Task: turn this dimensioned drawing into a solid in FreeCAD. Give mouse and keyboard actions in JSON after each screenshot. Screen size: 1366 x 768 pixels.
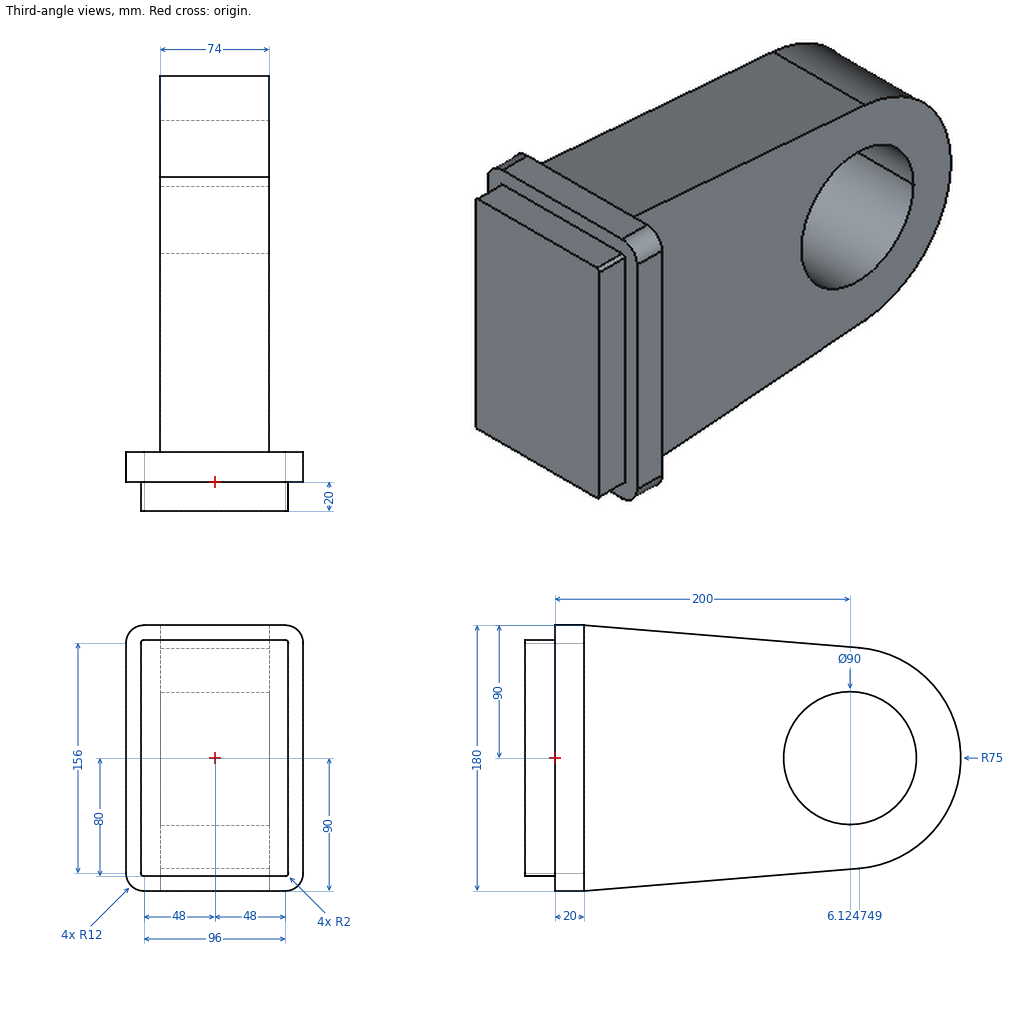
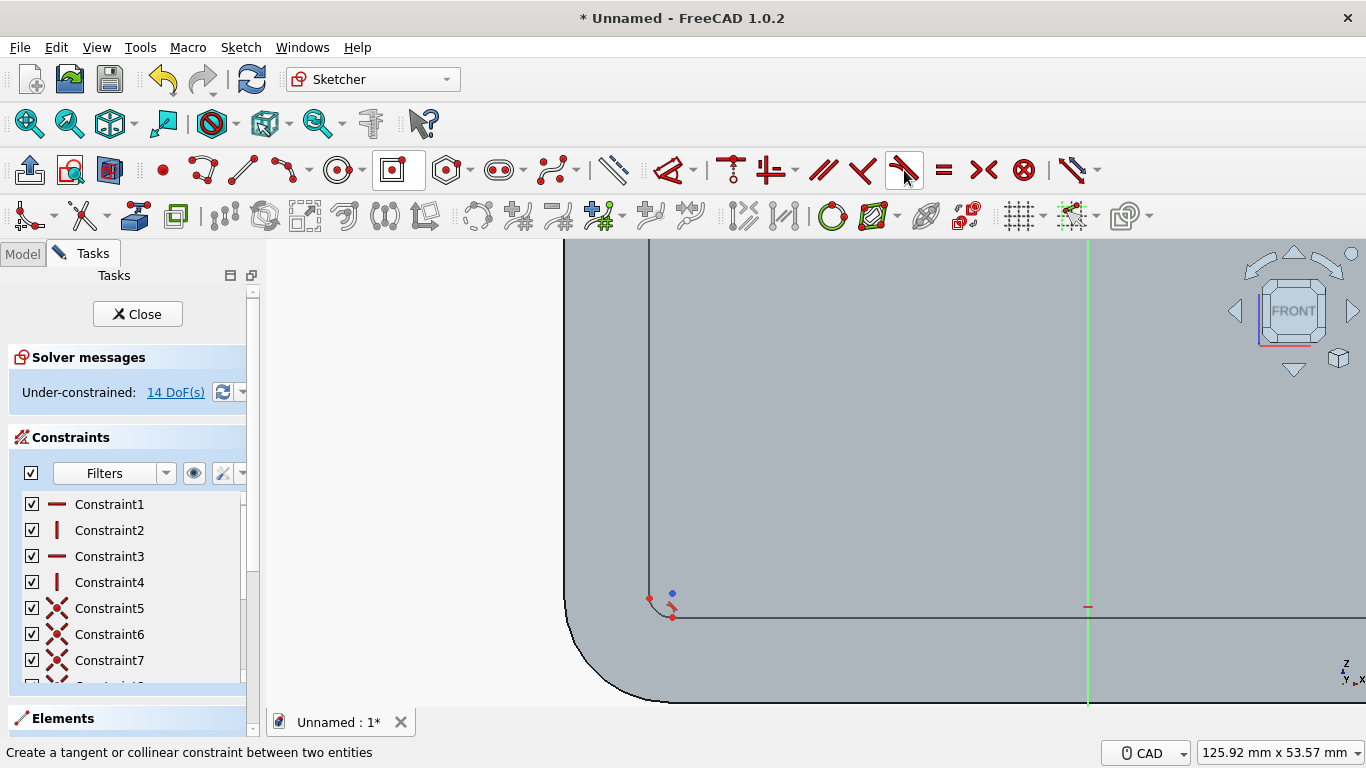
{"action": "scroll", "coordinate": [661, 614], "scroll_direction": "down", "scroll_amount": 8}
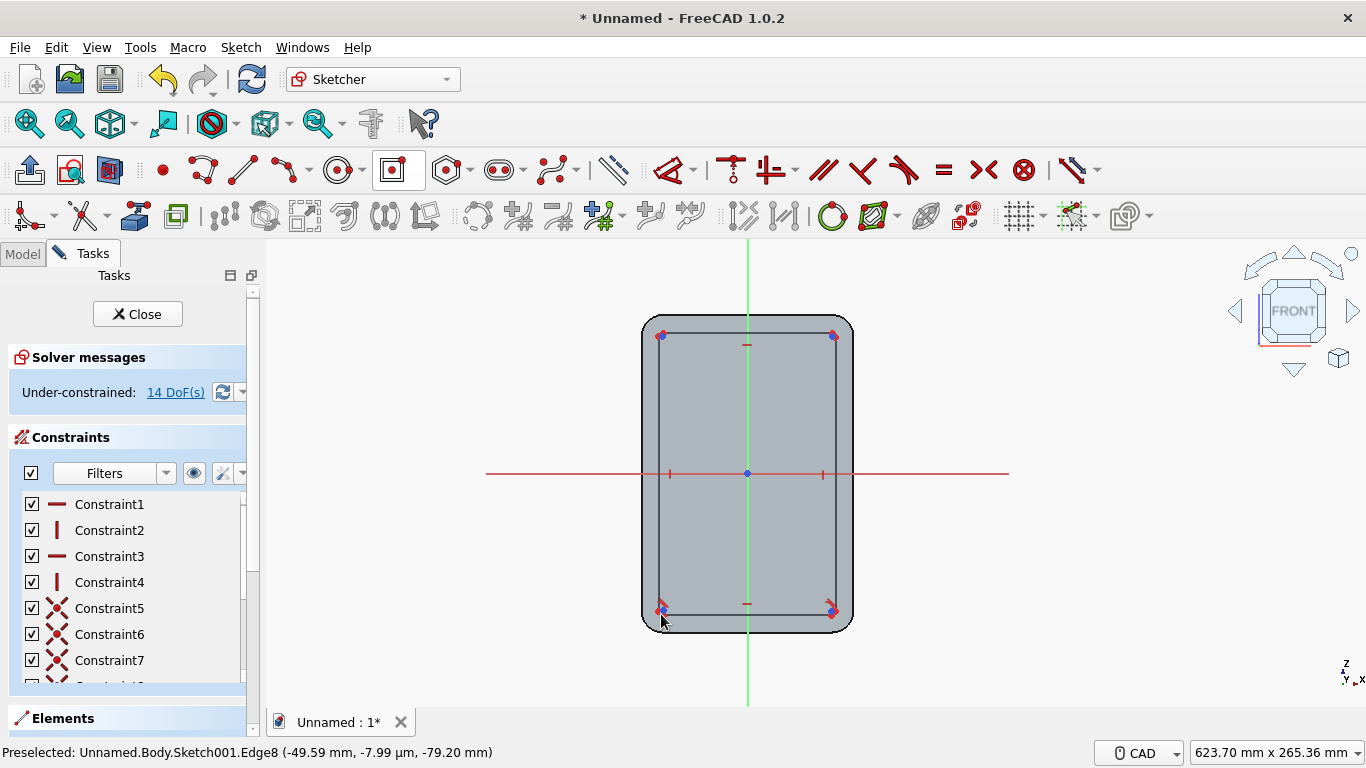
{"action": "left_click", "coordinate": [836, 529]}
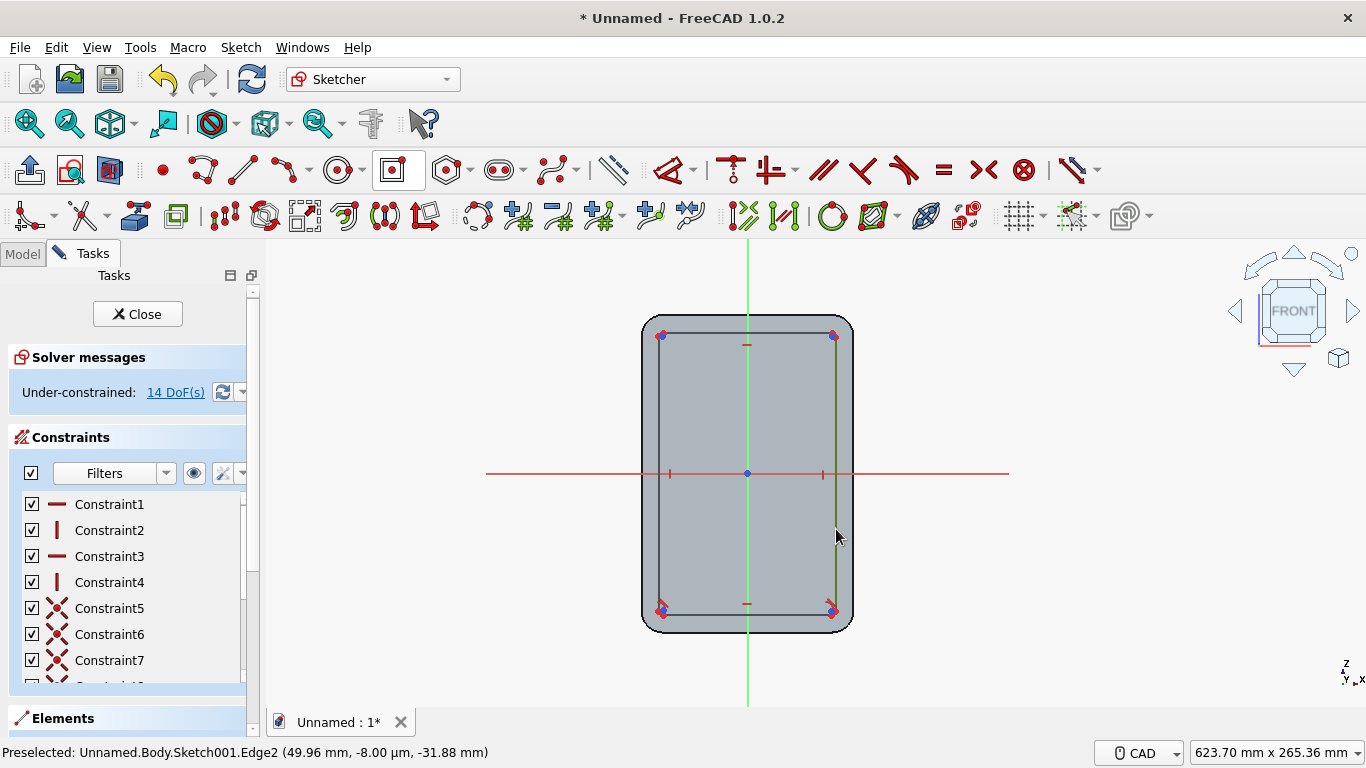
{"action": "scroll", "coordinate": [834, 614], "scroll_direction": "up", "scroll_amount": 8}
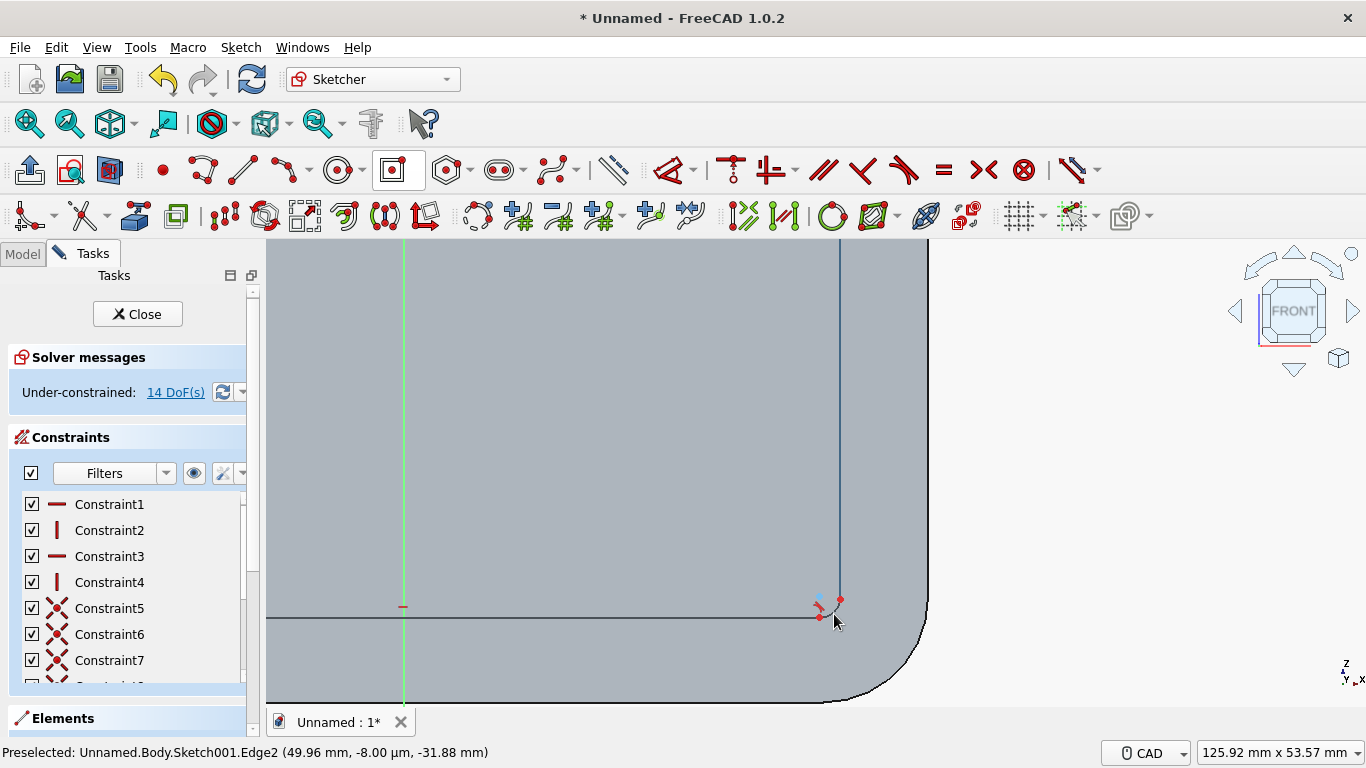
{"action": "left_click", "coordinate": [833, 613]}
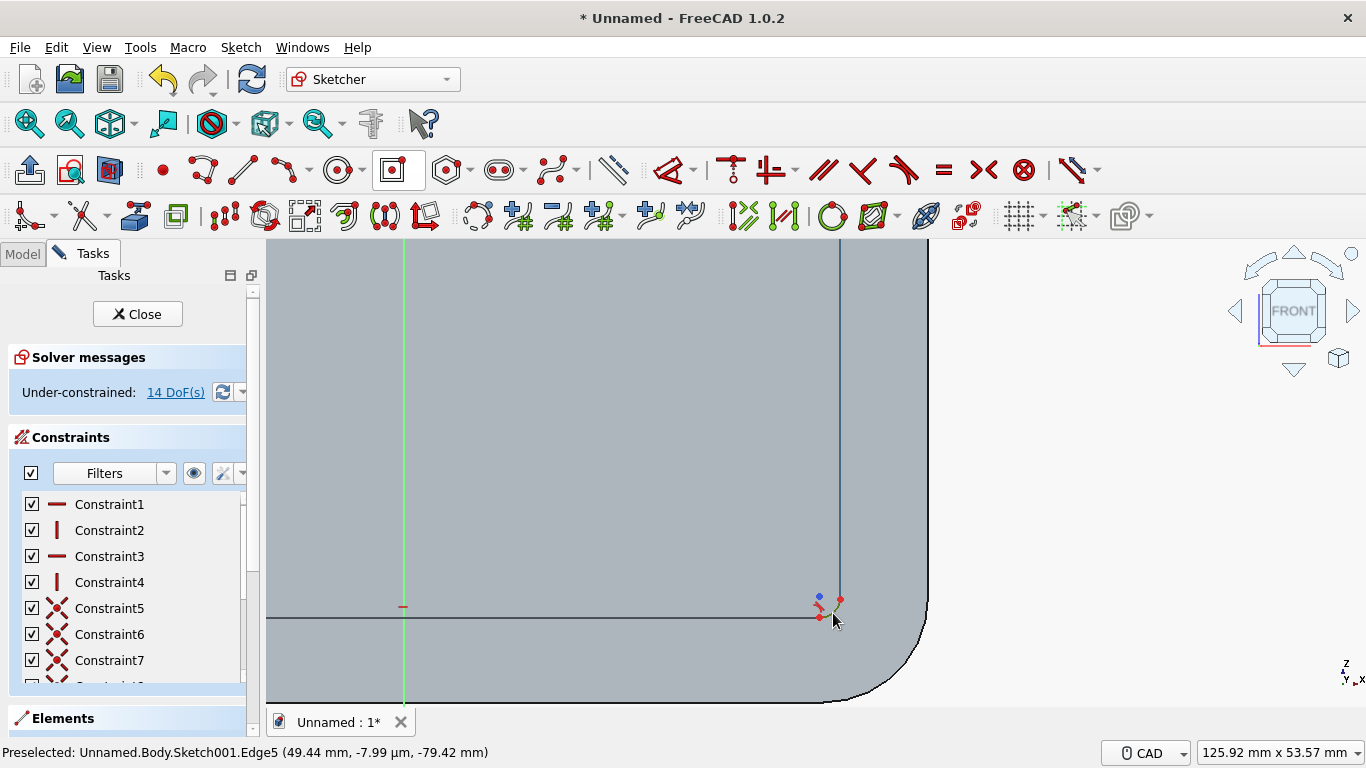
{"action": "key", "text": "t"}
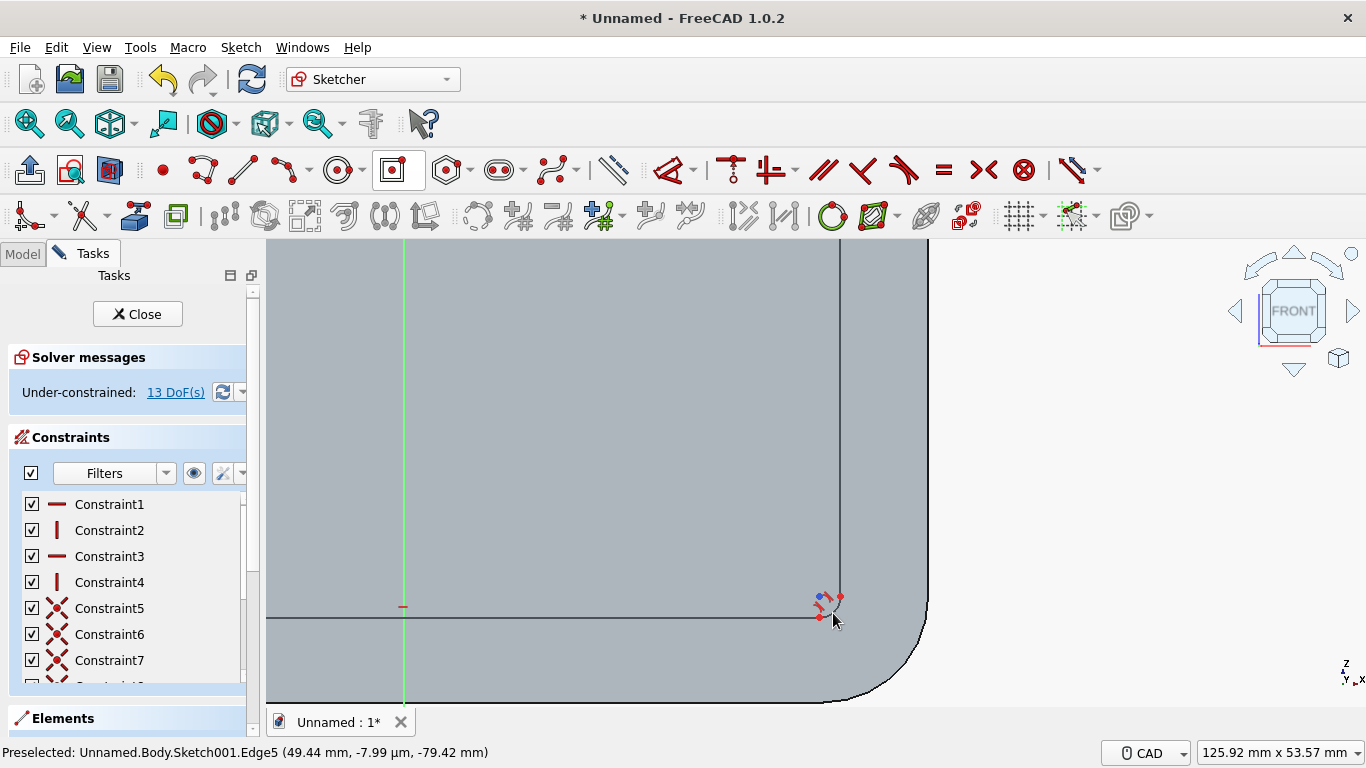
{"action": "scroll", "coordinate": [834, 614], "scroll_direction": "down", "scroll_amount": 8}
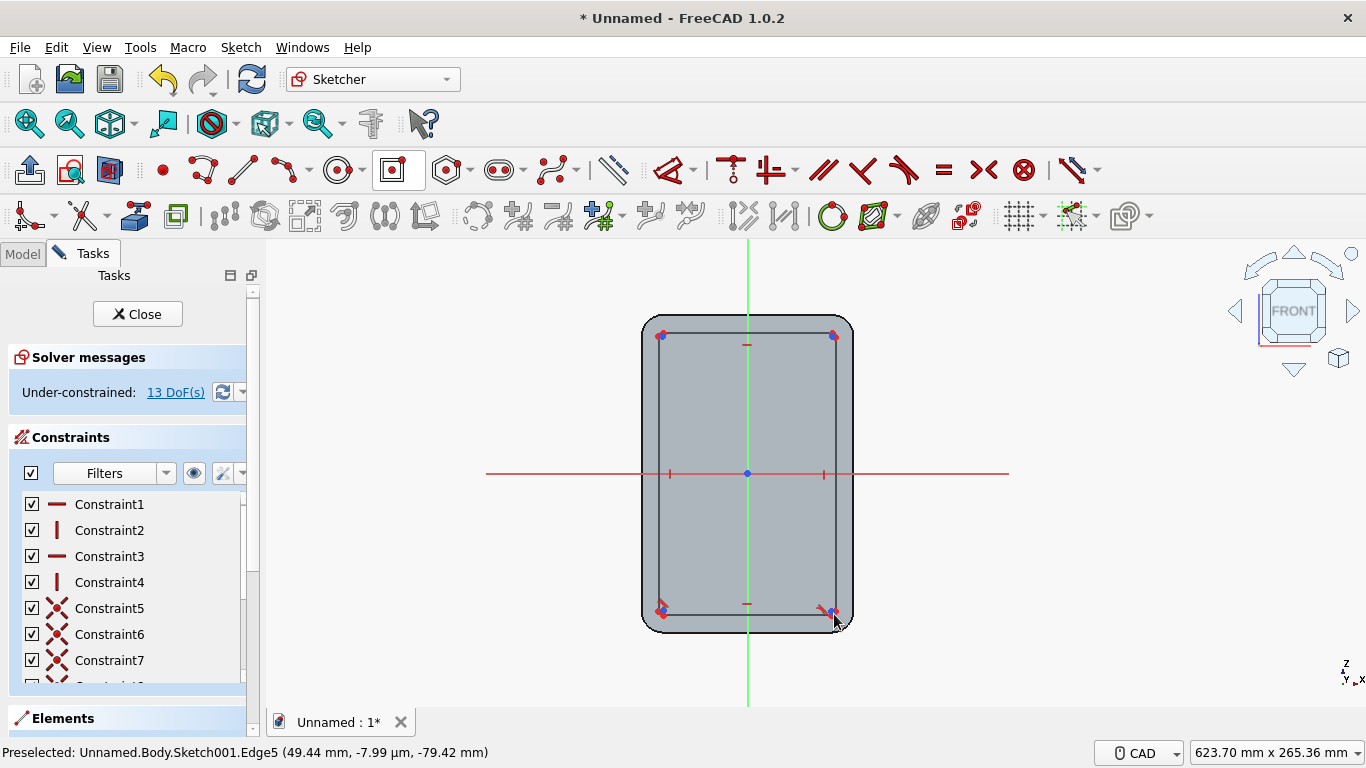
{"action": "left_click", "coordinate": [836, 556]}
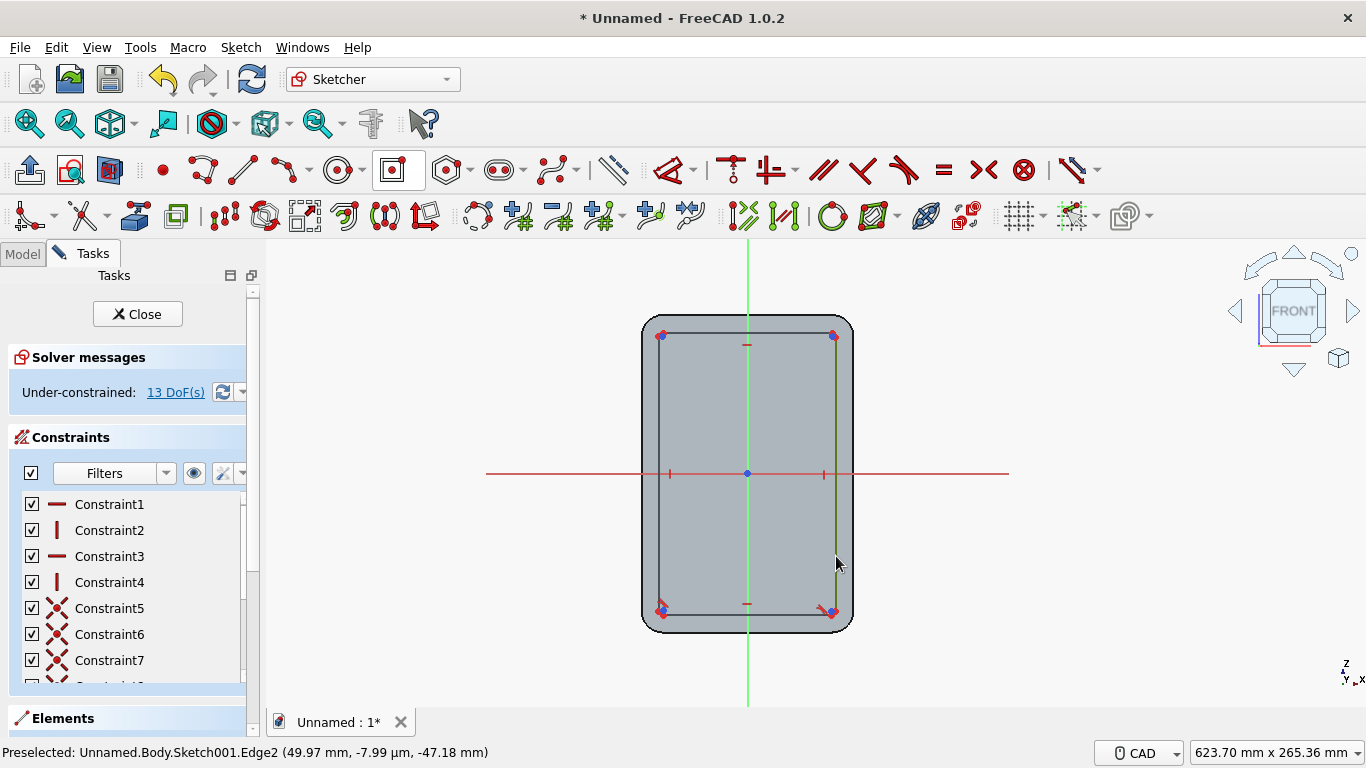
{"action": "scroll", "coordinate": [835, 334], "scroll_direction": "up", "scroll_amount": 8}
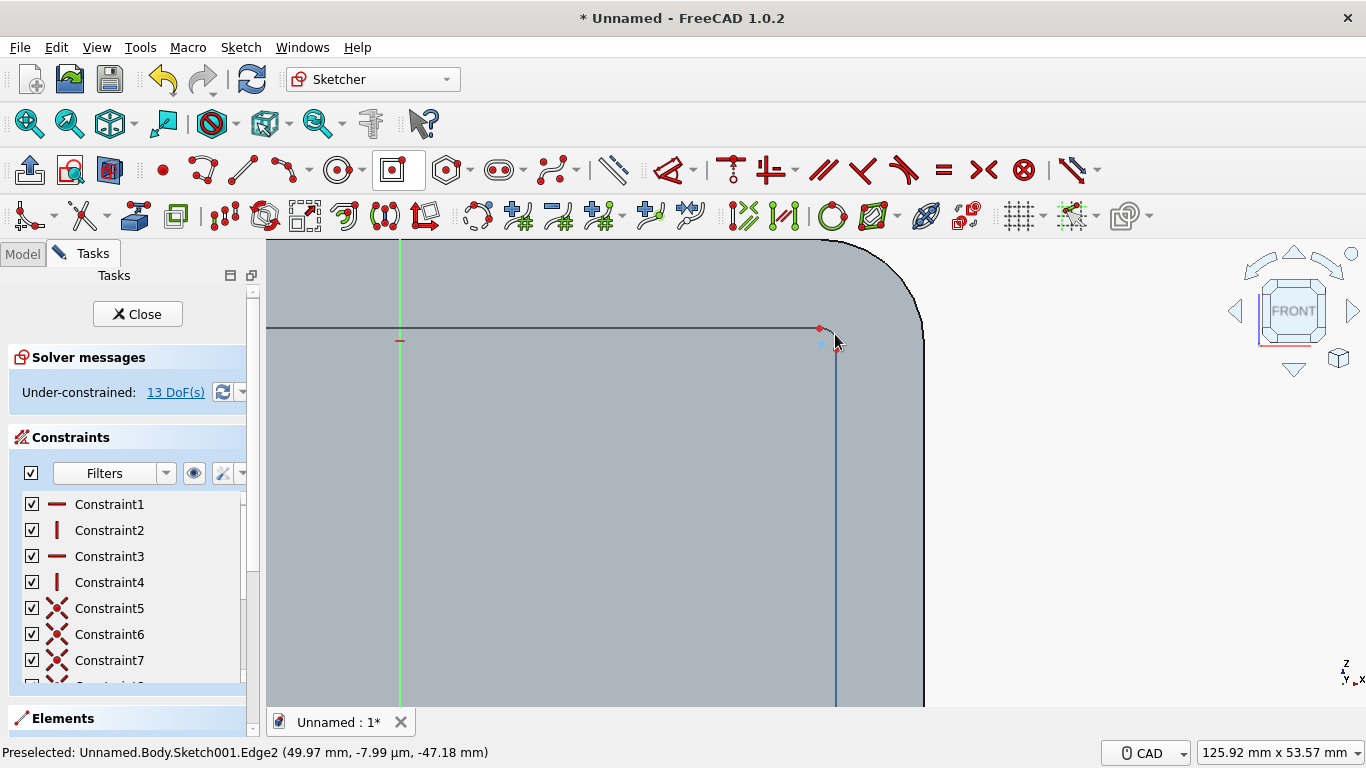
{"action": "left_click", "coordinate": [834, 334]}